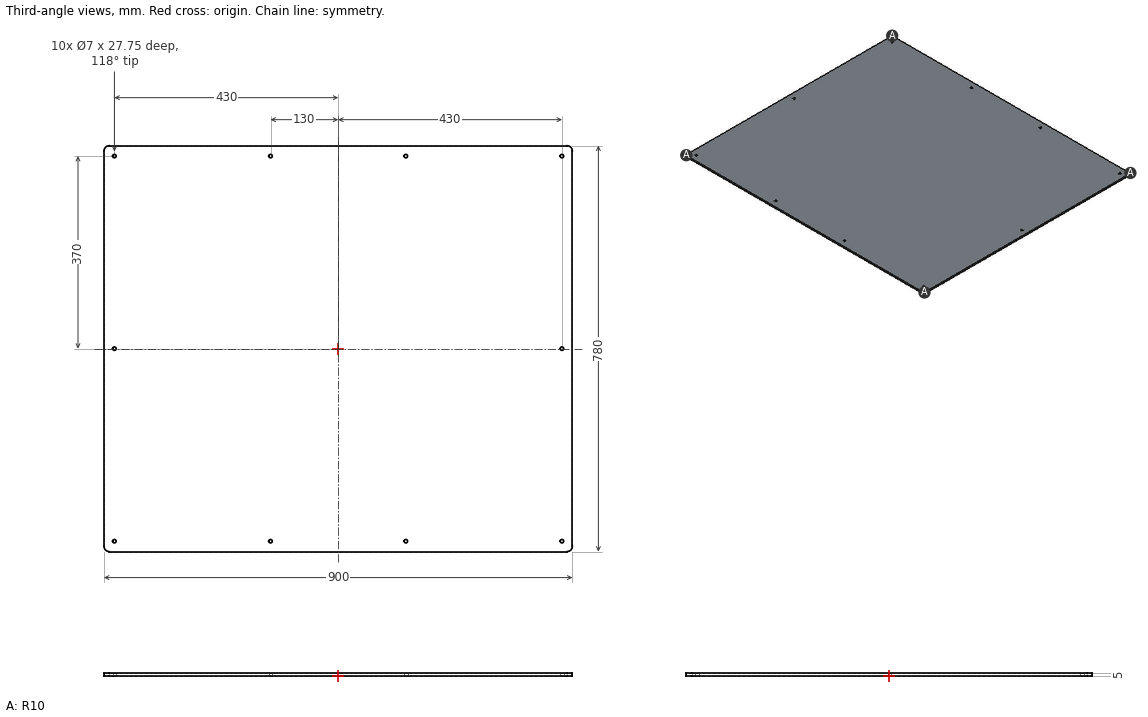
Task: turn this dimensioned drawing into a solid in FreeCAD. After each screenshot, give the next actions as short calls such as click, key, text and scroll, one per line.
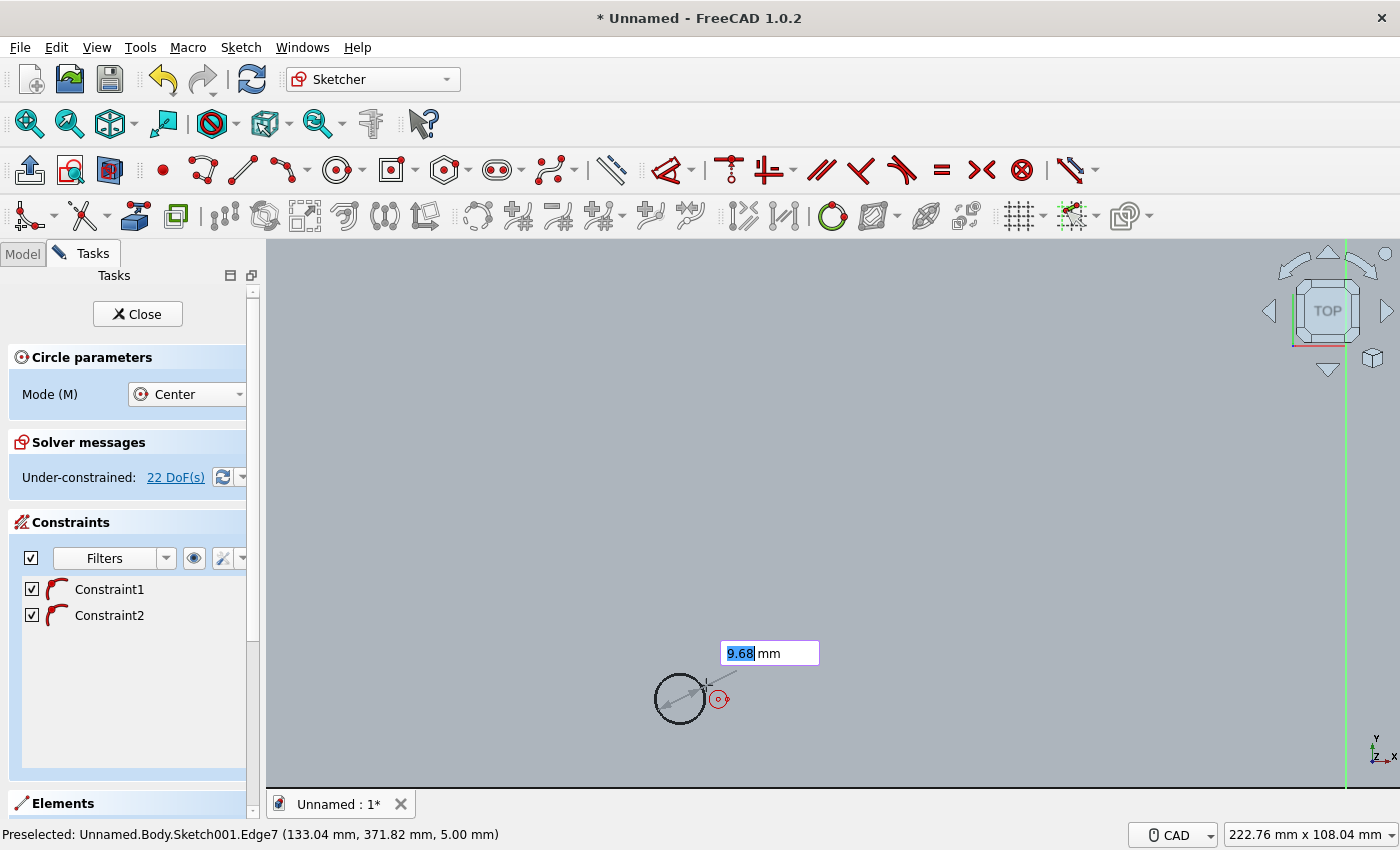
click(697, 674)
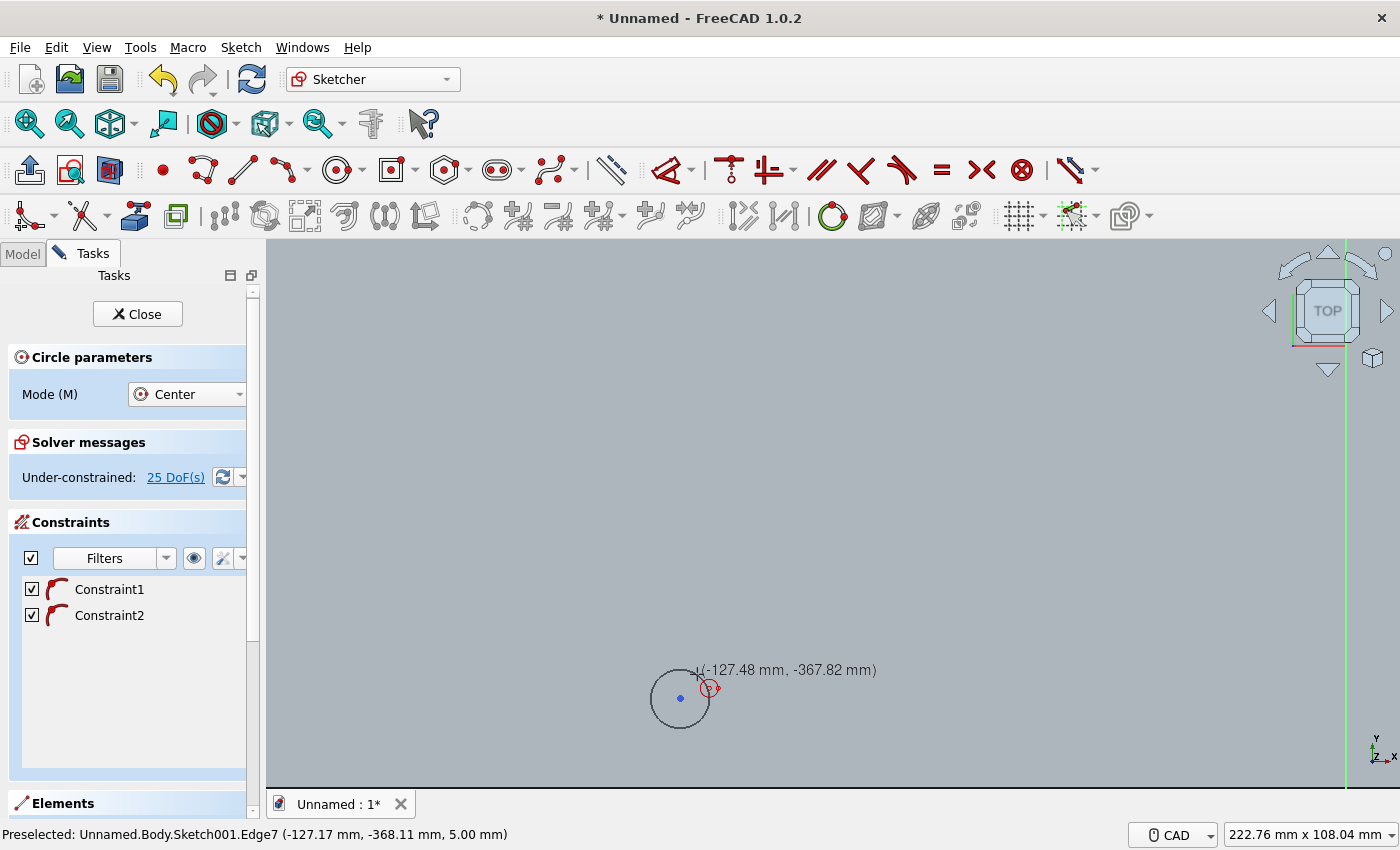
scroll(706, 685, down, 12)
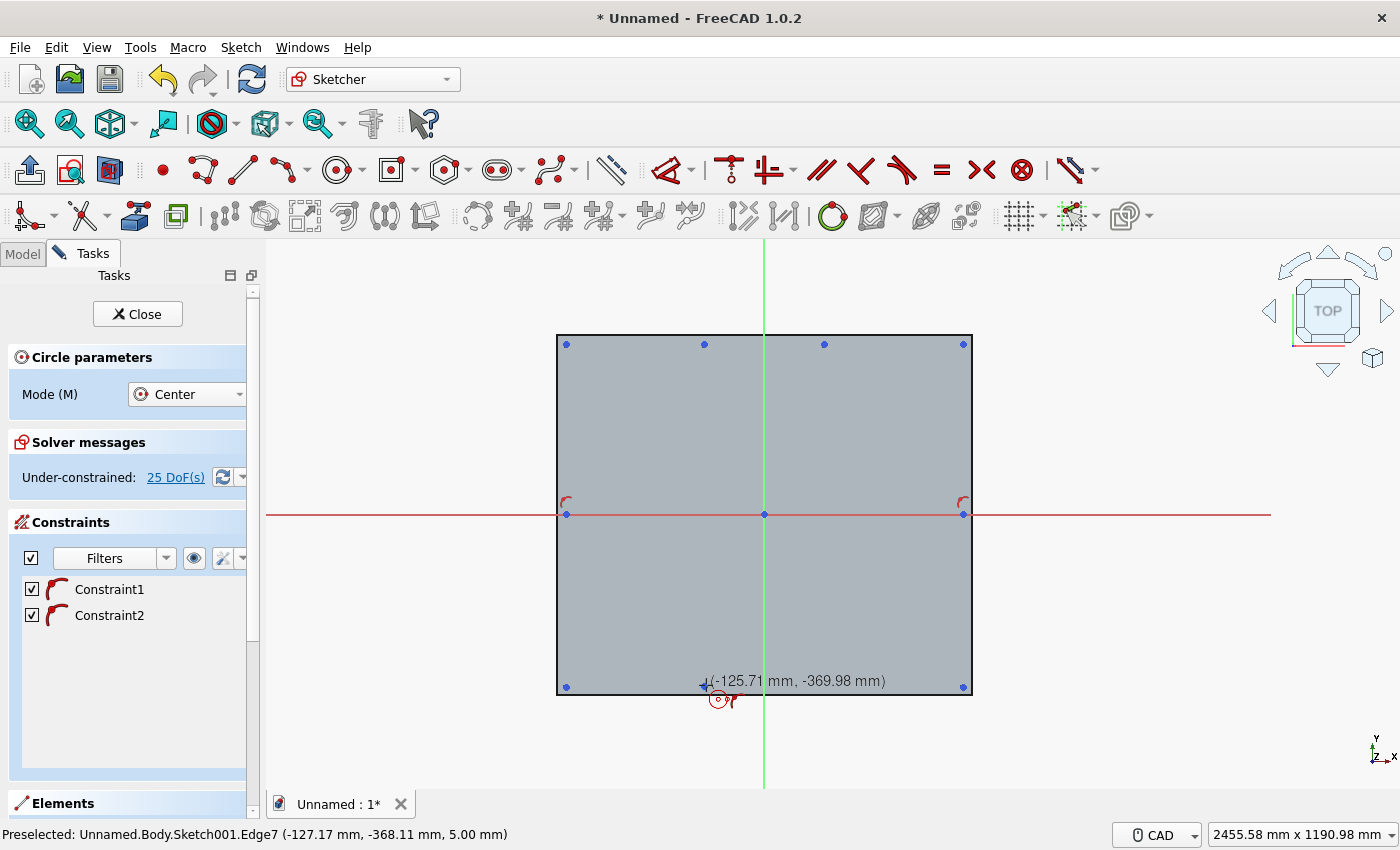
scroll(824, 686, up, 14)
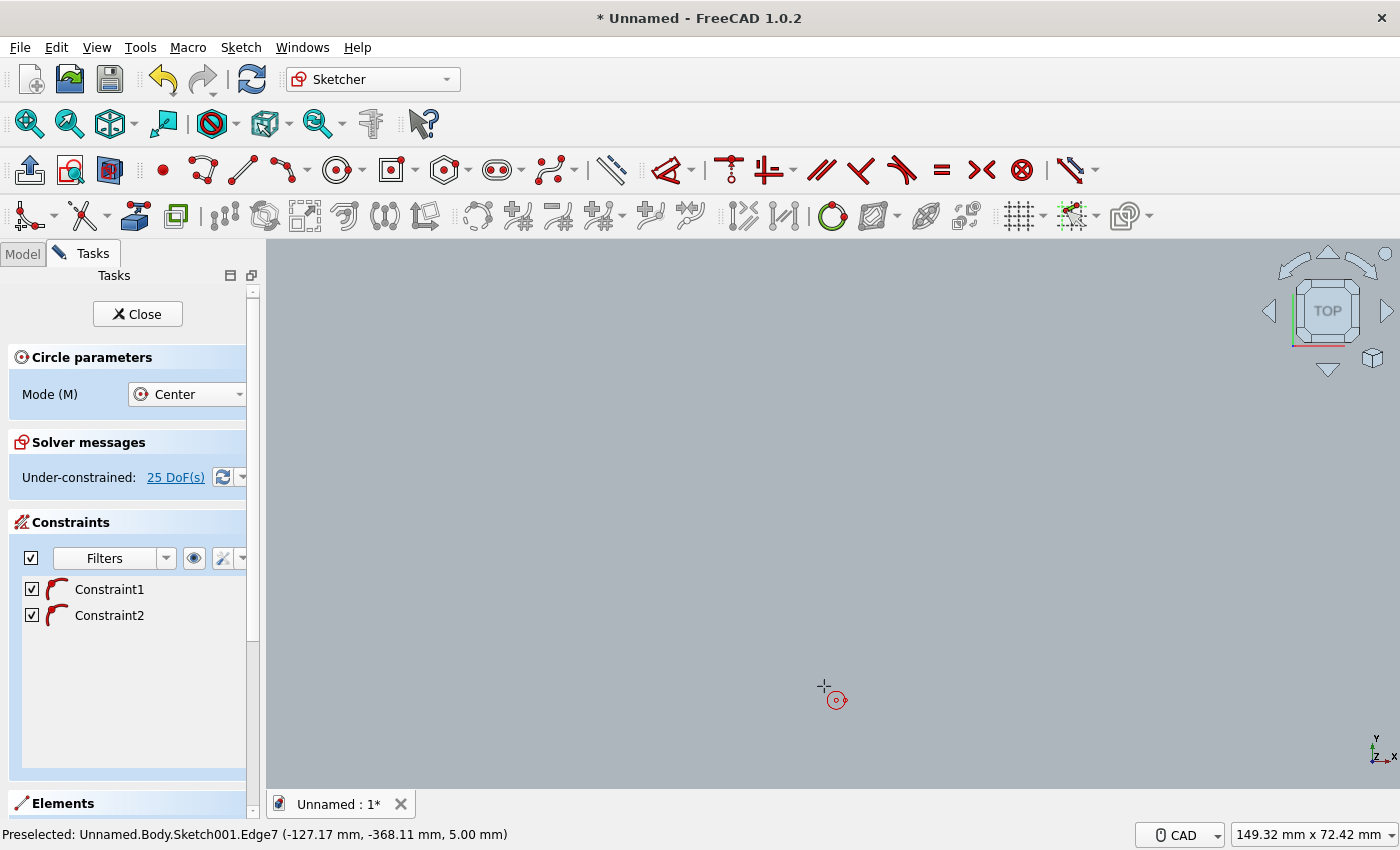
scroll(825, 686, down, 14)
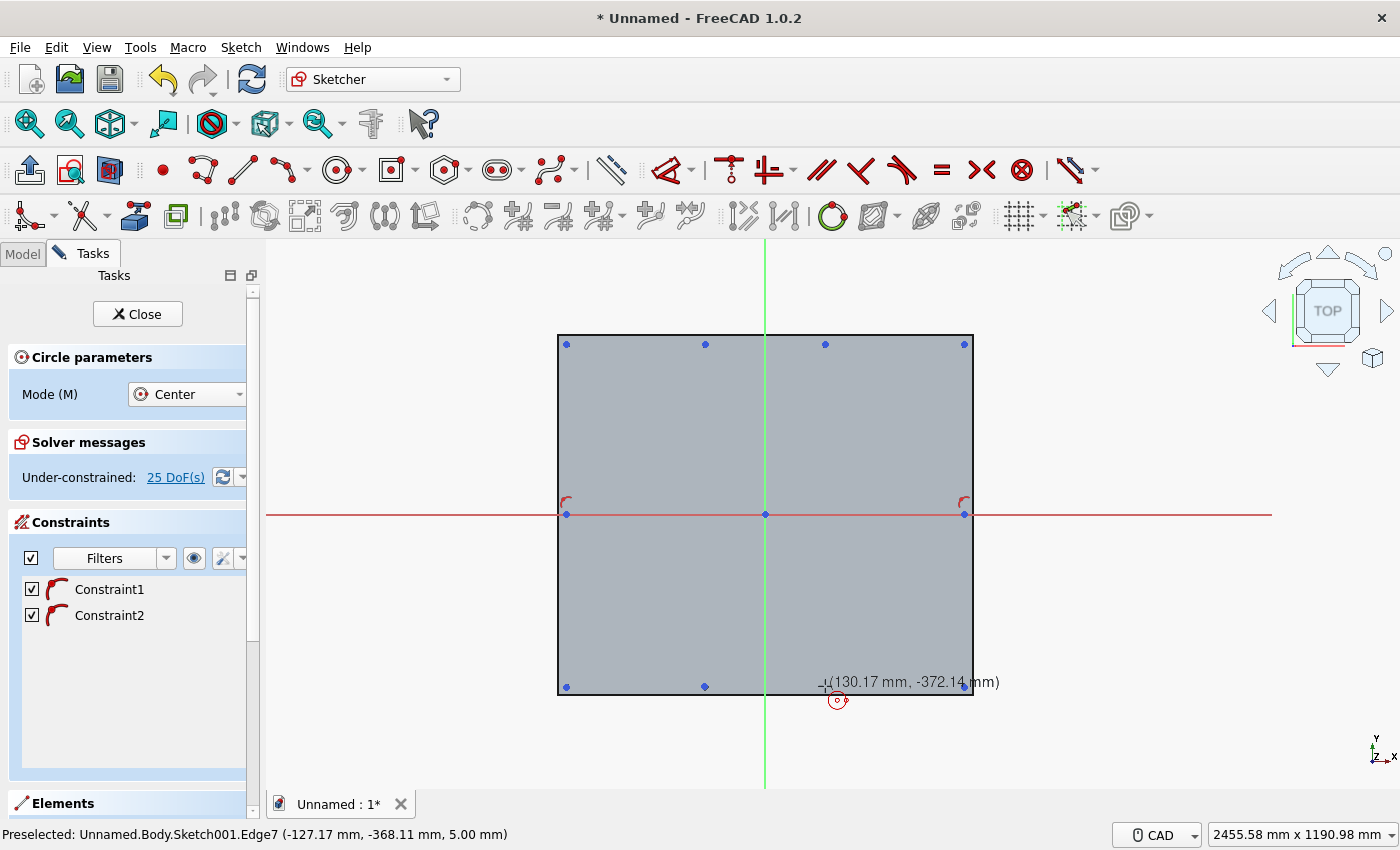
click(825, 686)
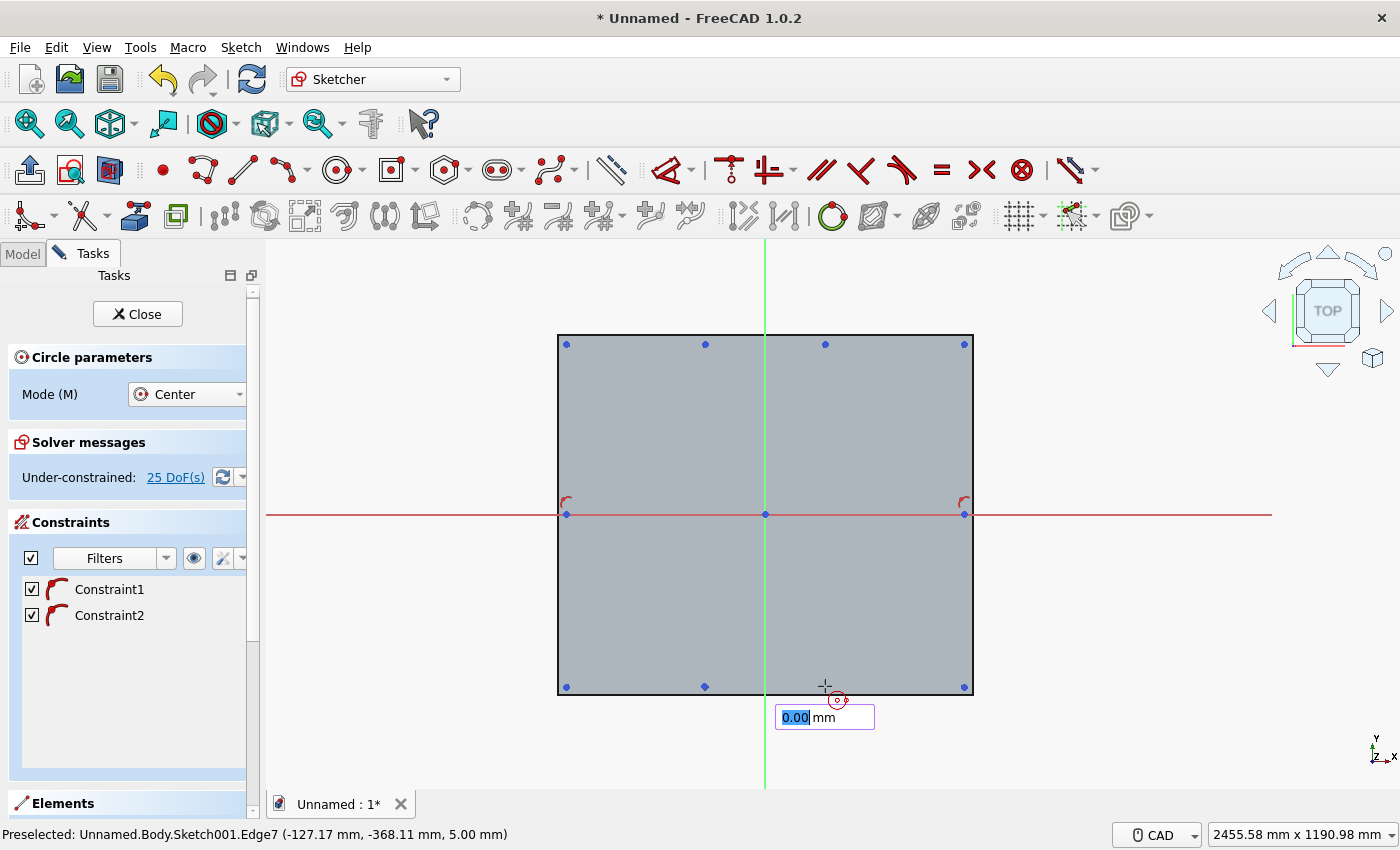
scroll(827, 685, up, 12)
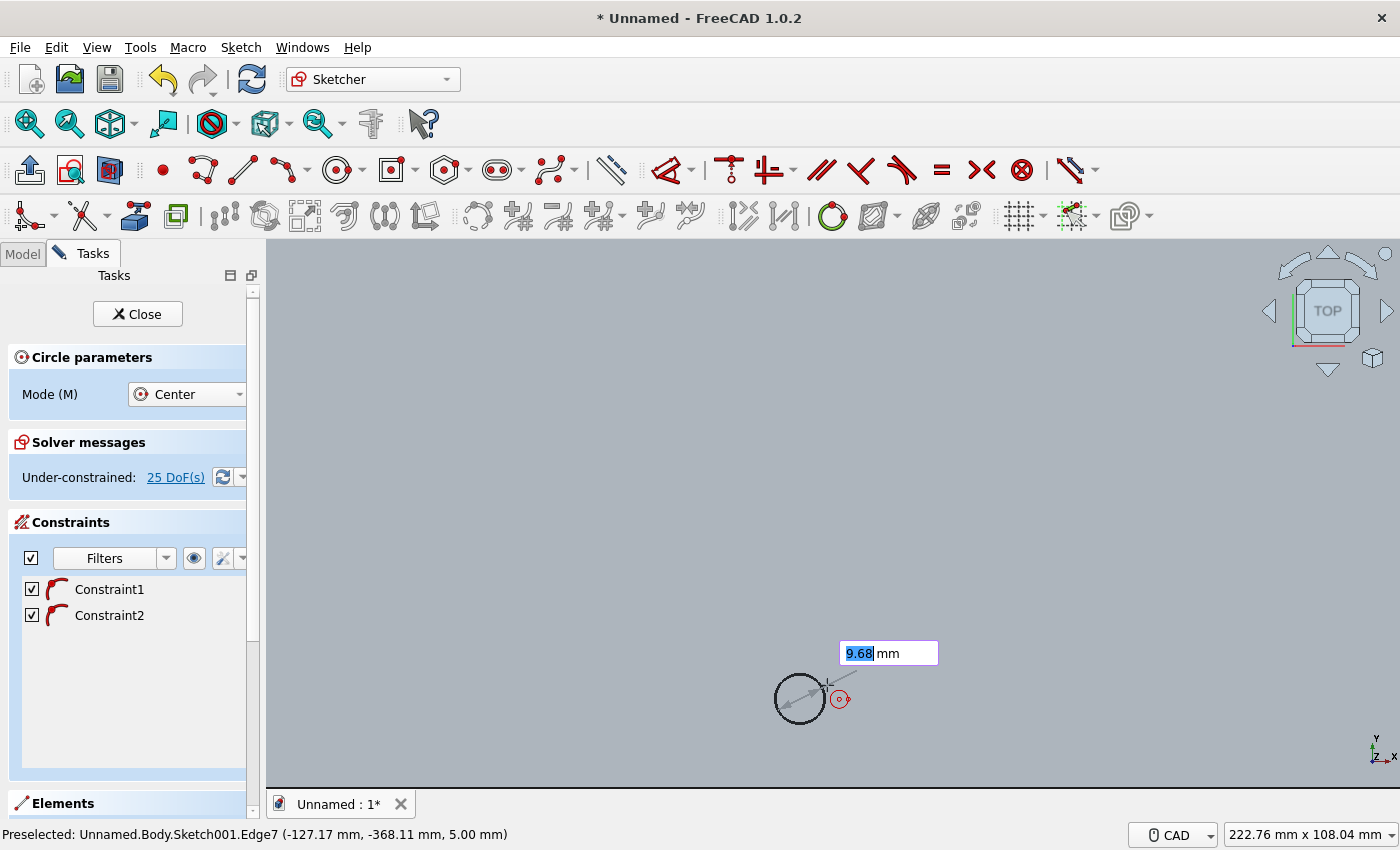
click(817, 674)
key(Escape)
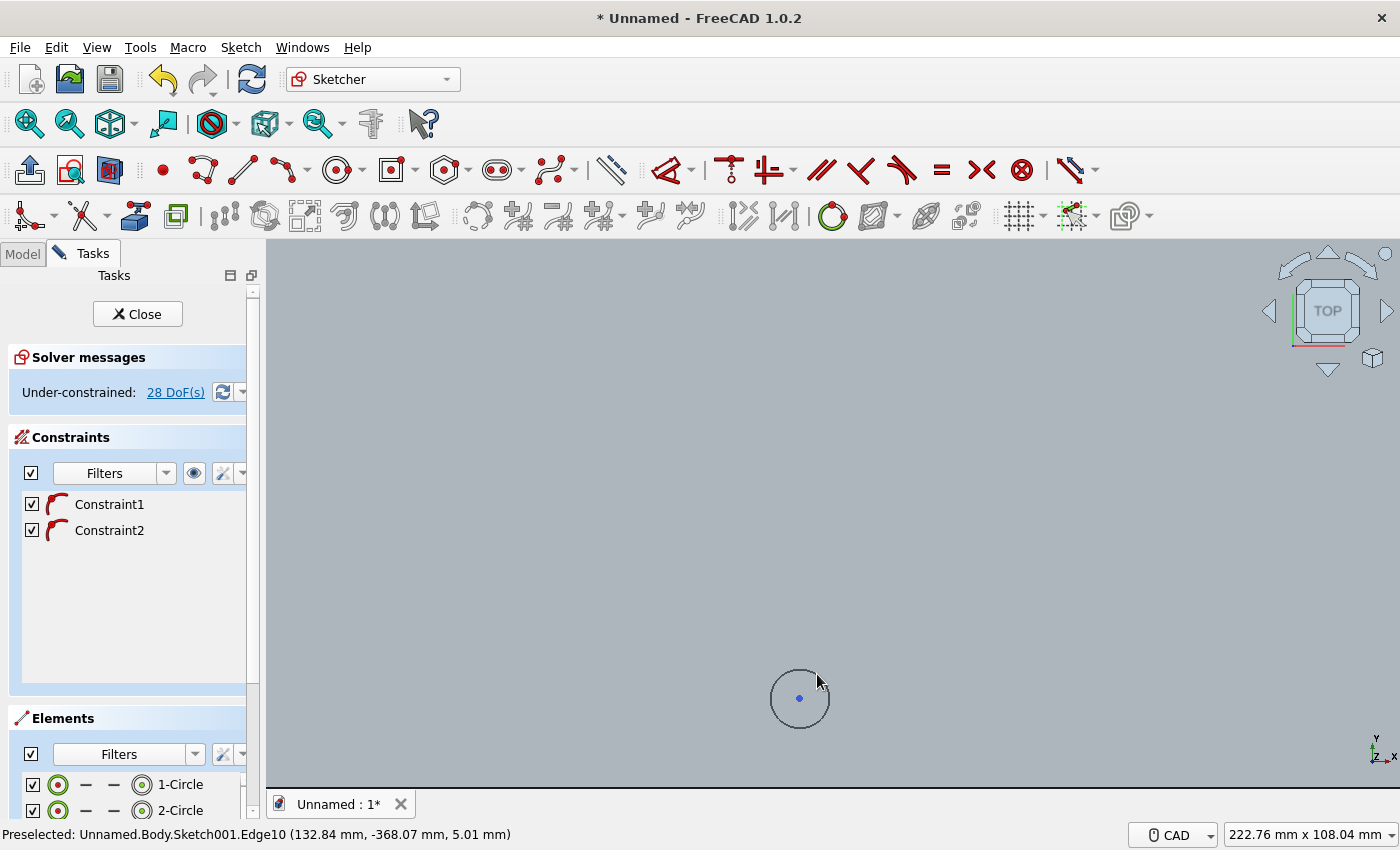
scroll(827, 685, down, 12)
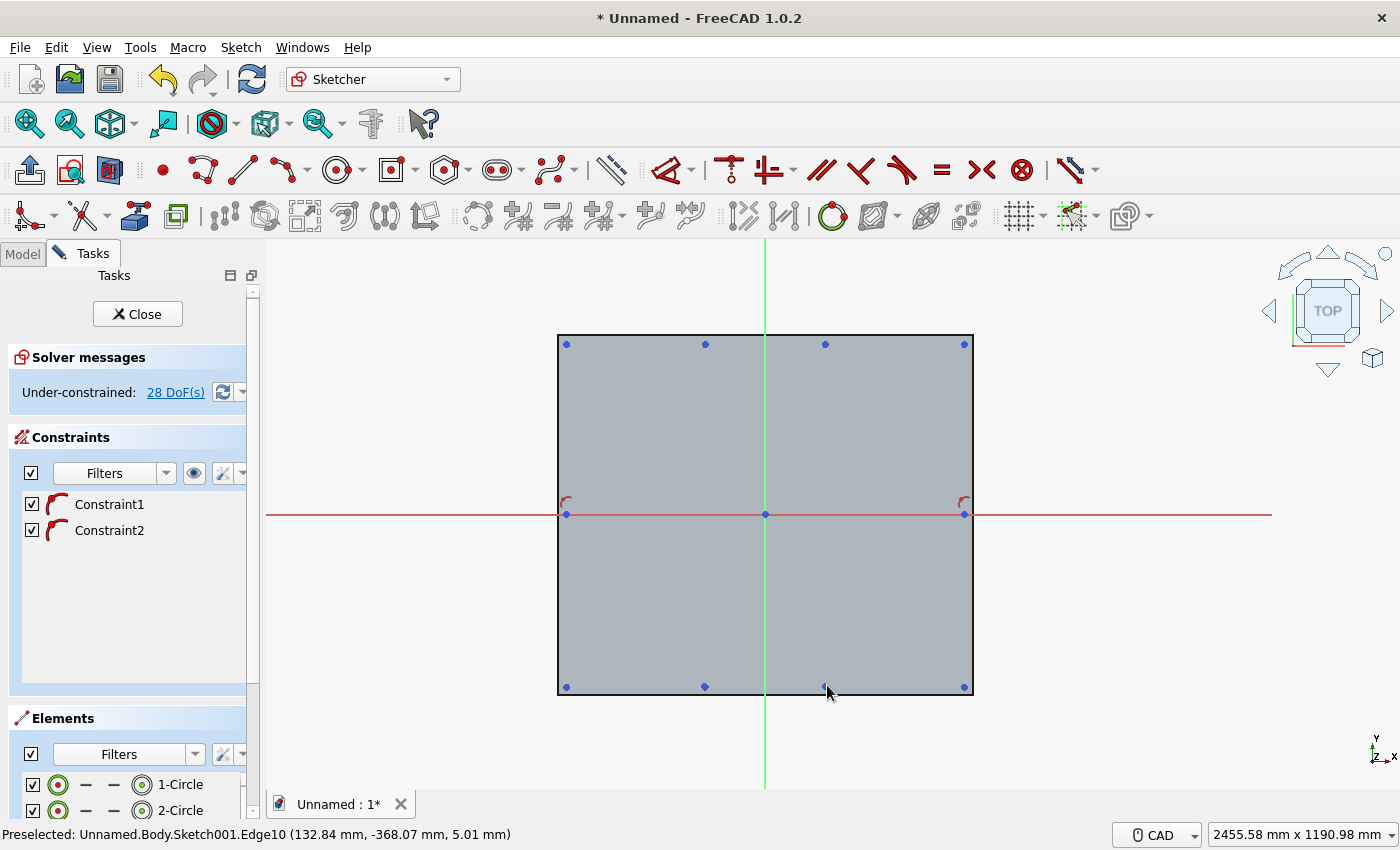
scroll(568, 343, up, 10)